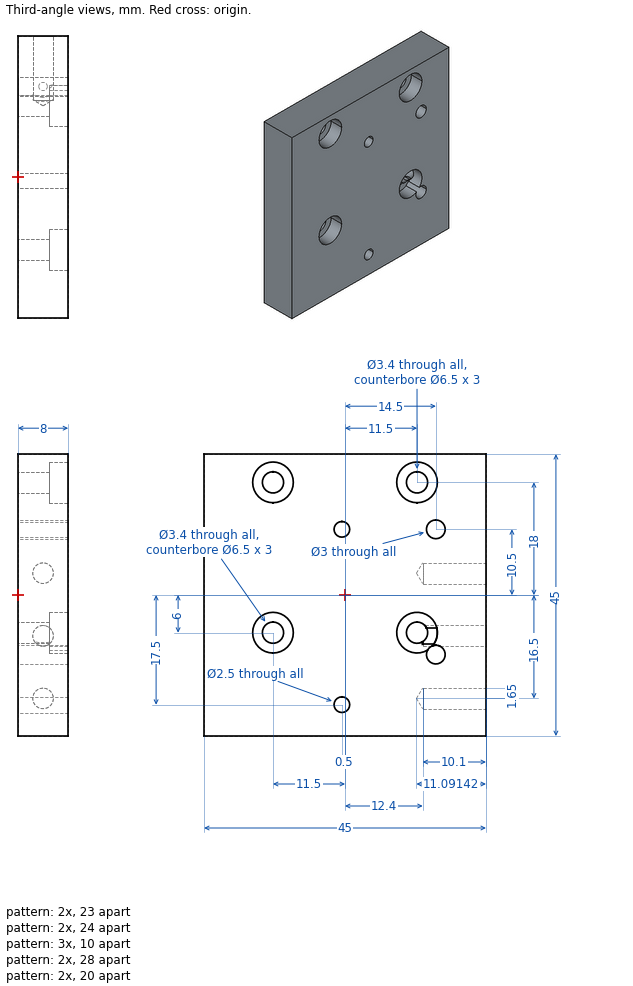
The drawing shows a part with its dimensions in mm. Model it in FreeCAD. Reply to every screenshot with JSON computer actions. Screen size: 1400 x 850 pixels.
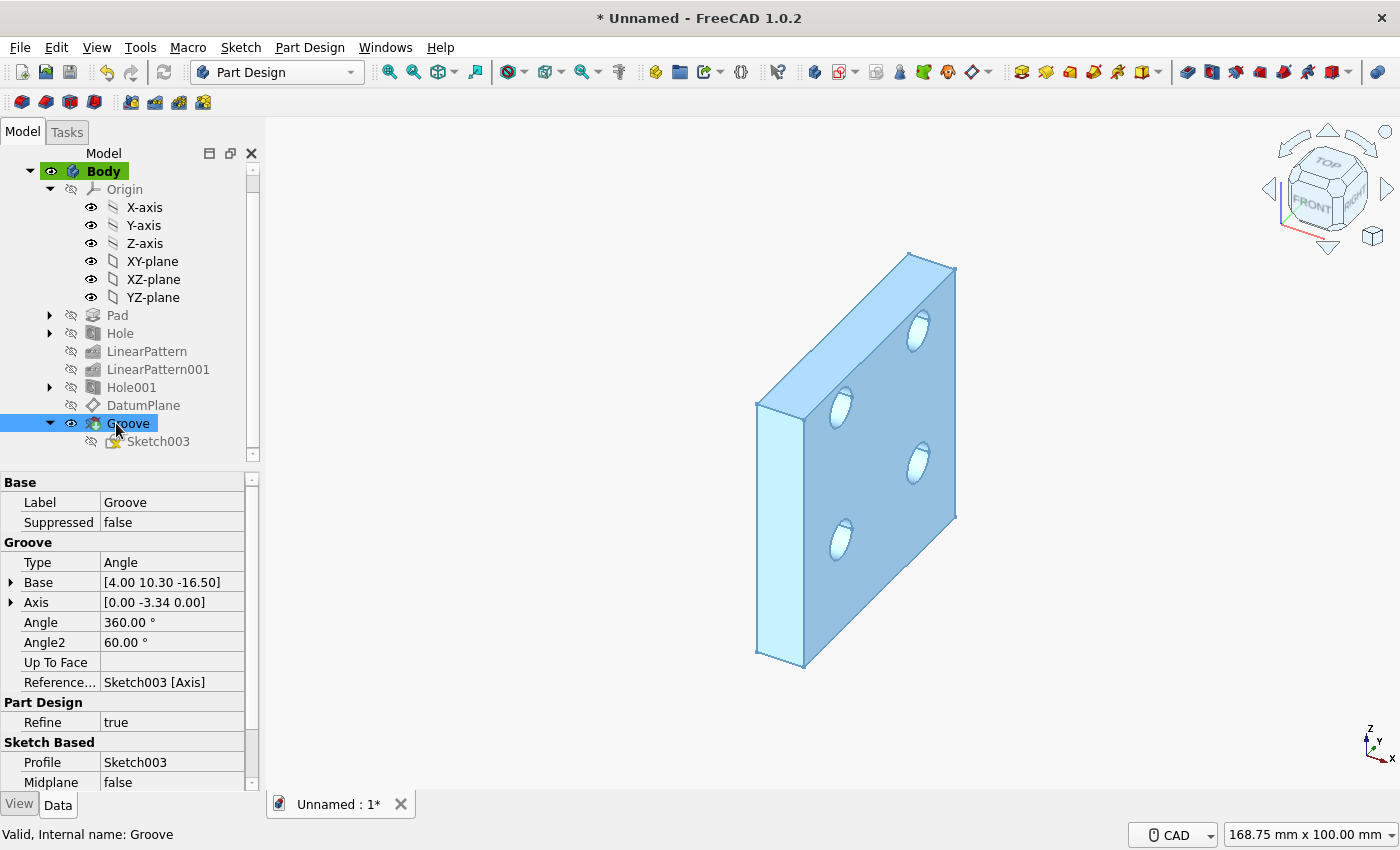
{"action": "left_click", "coordinate": [156, 102]}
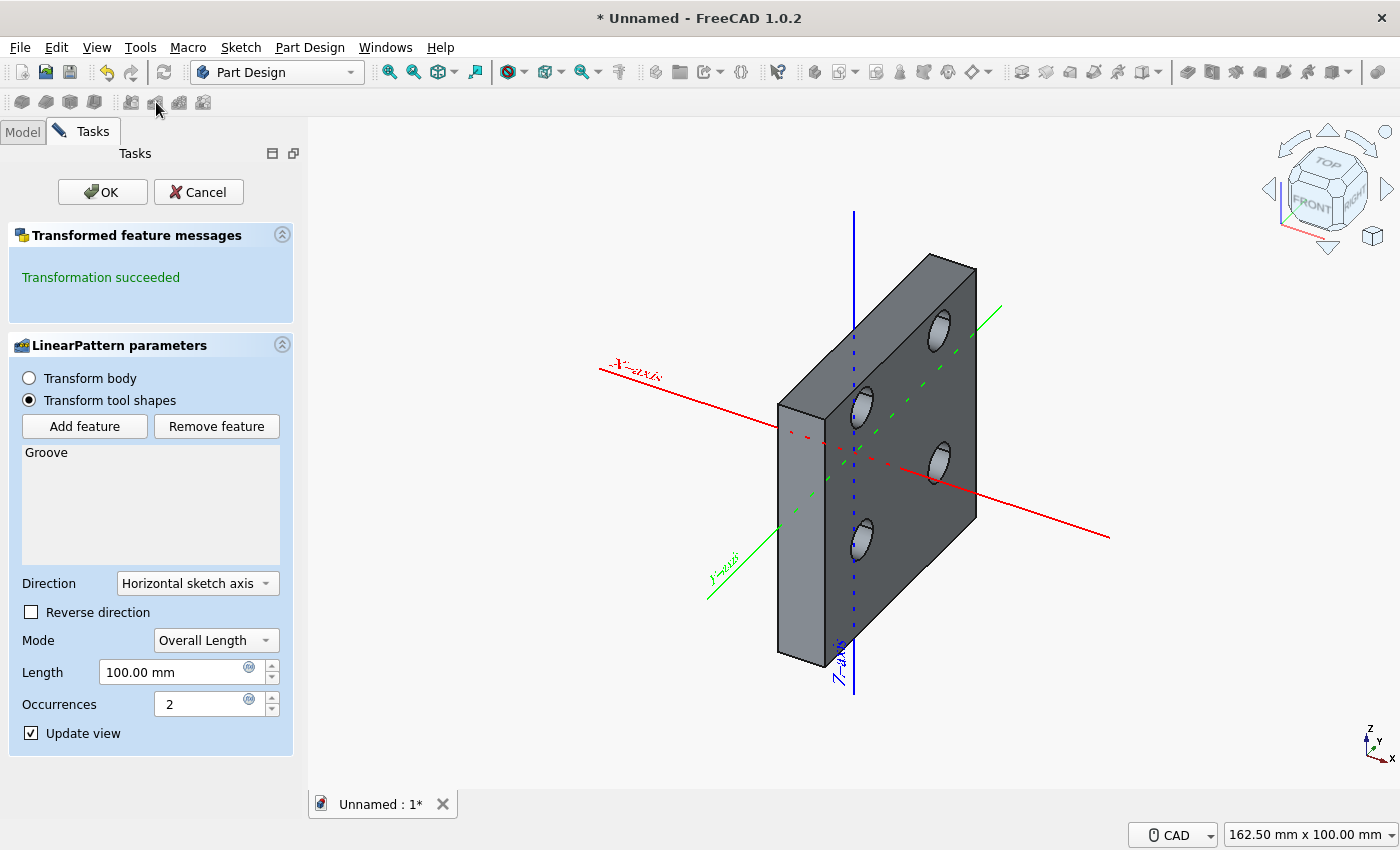
{"action": "left_click", "coordinate": [198, 584]}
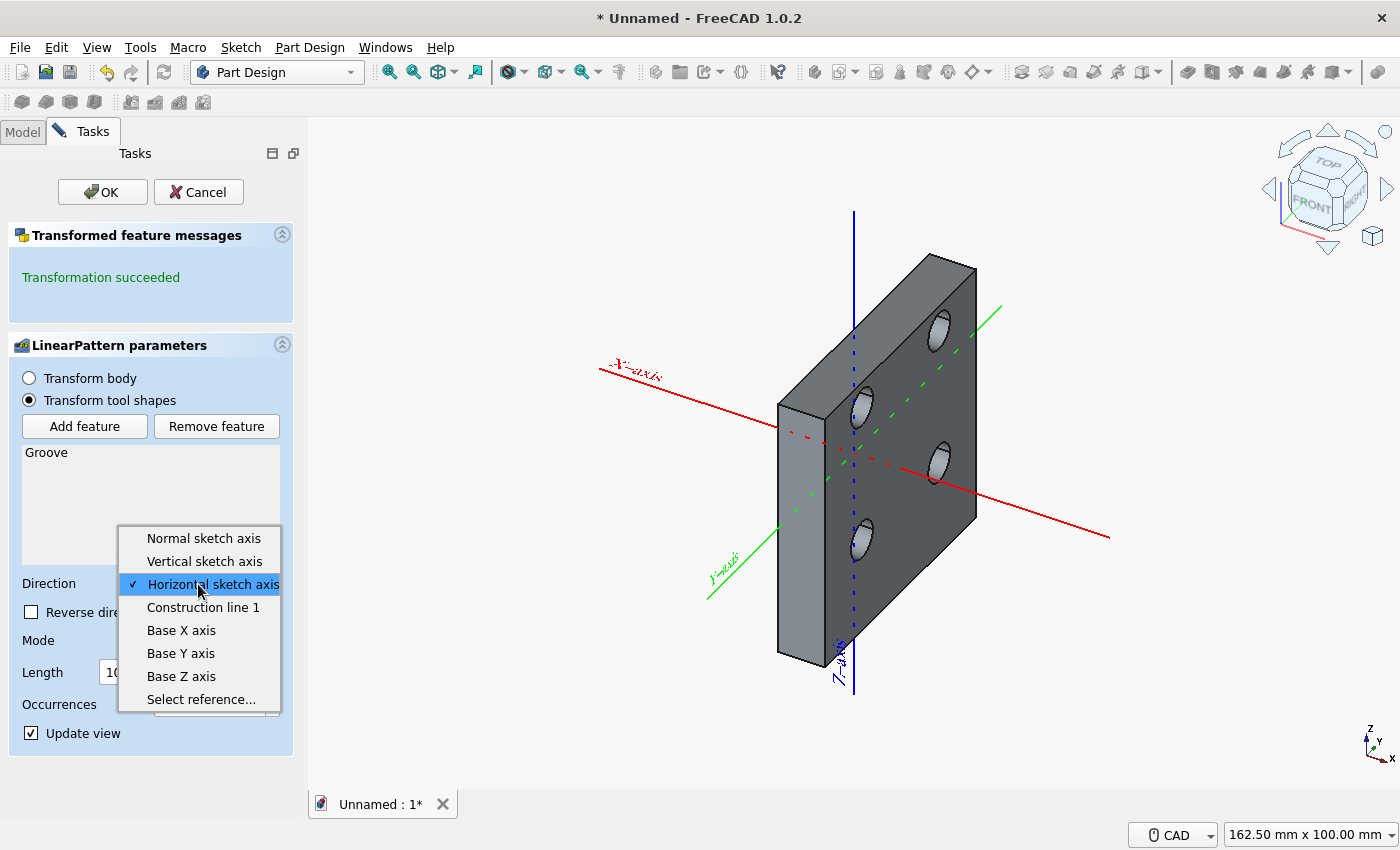
{"action": "left_click", "coordinate": [198, 676]}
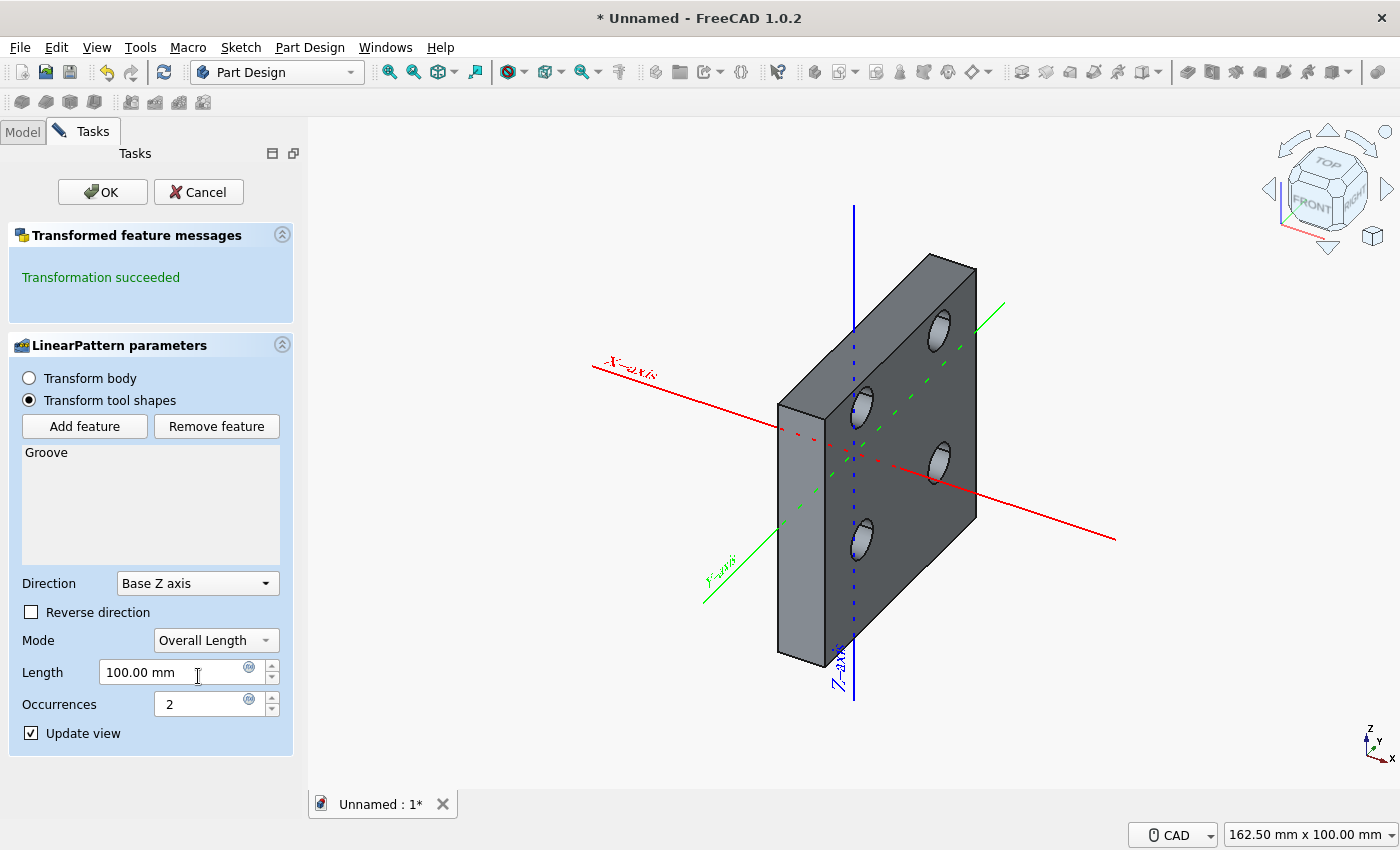
{"action": "left_click", "coordinate": [217, 640]}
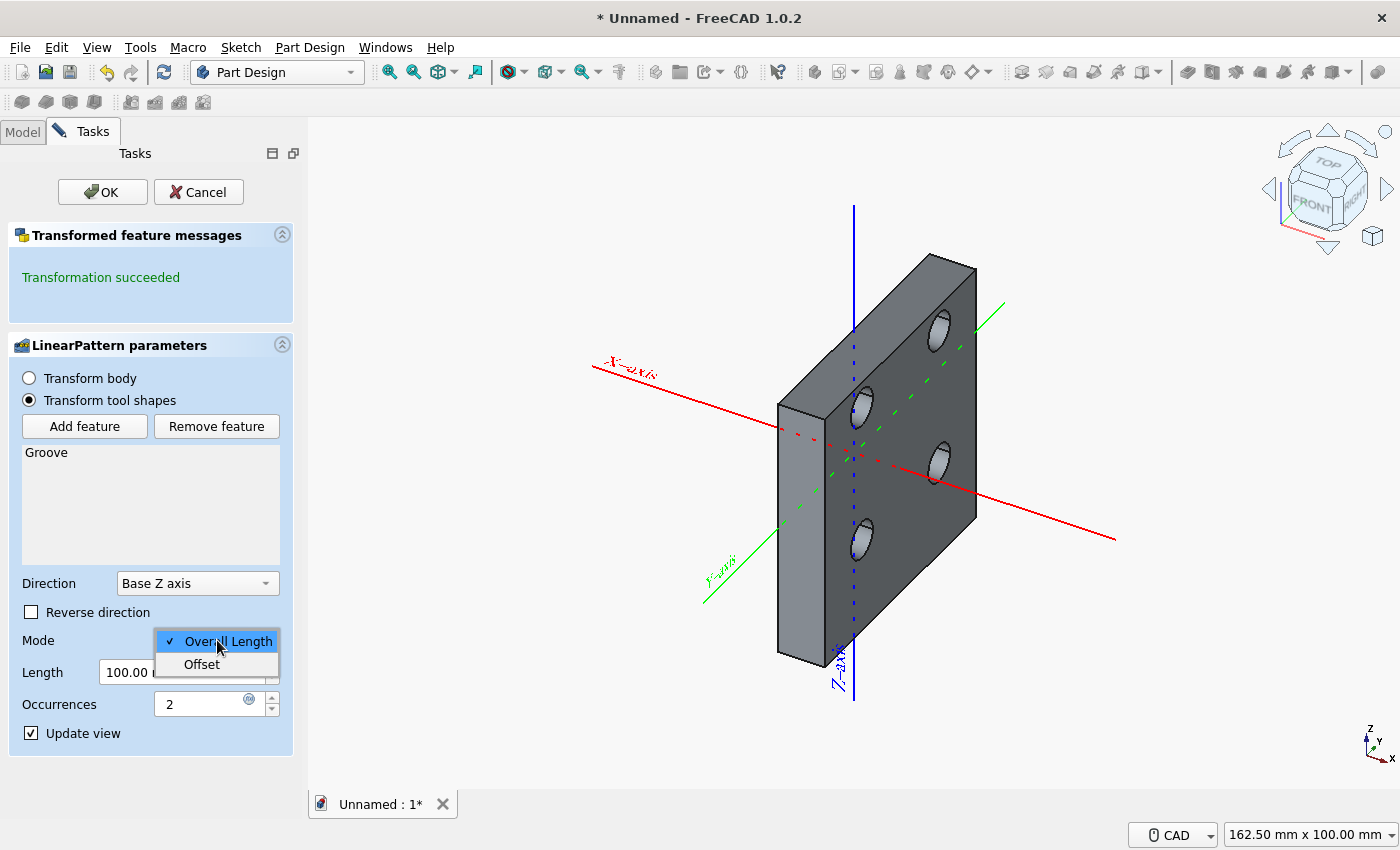
{"action": "left_click", "coordinate": [216, 664]}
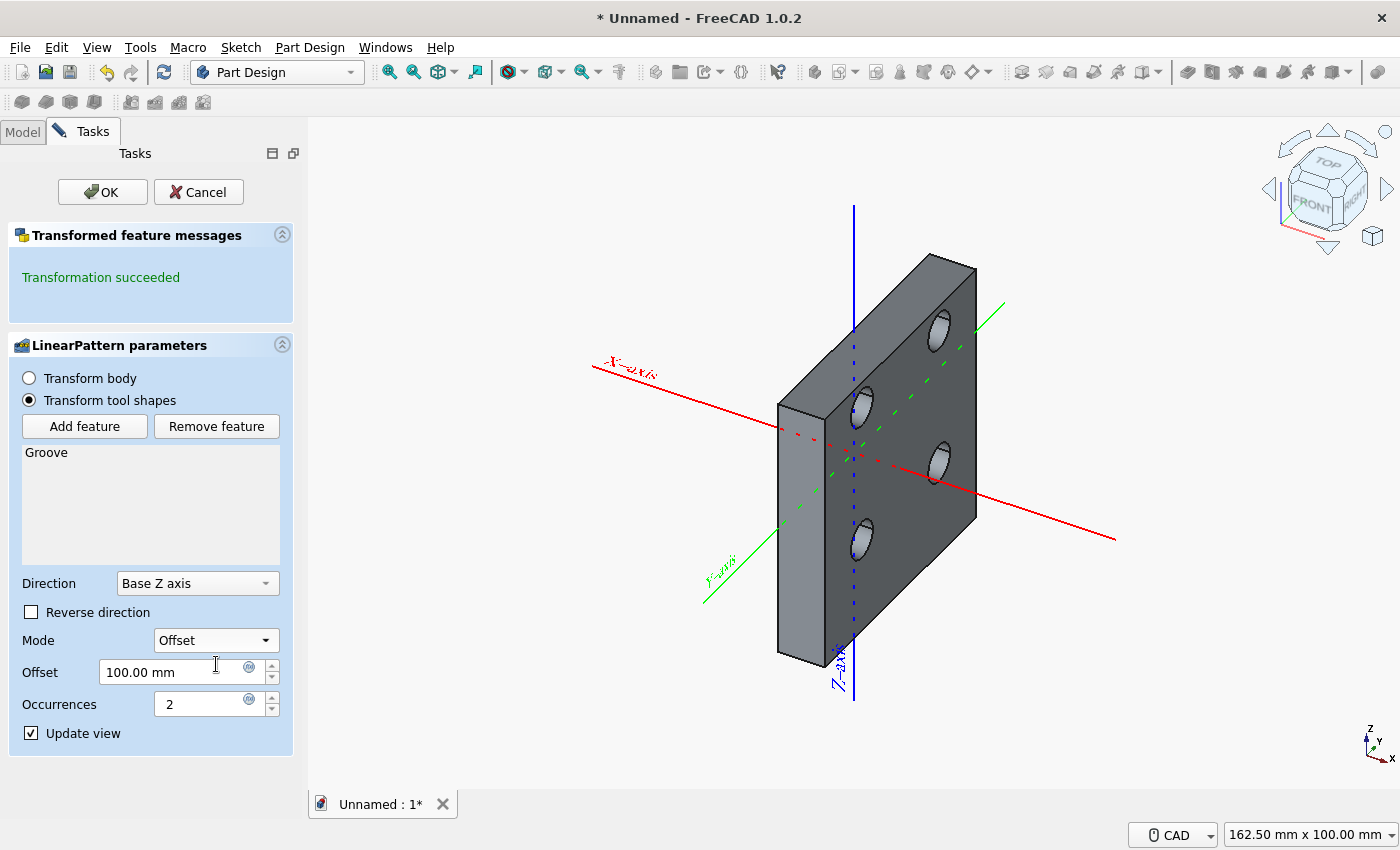
{"action": "triple_click", "coordinate": [182, 672]}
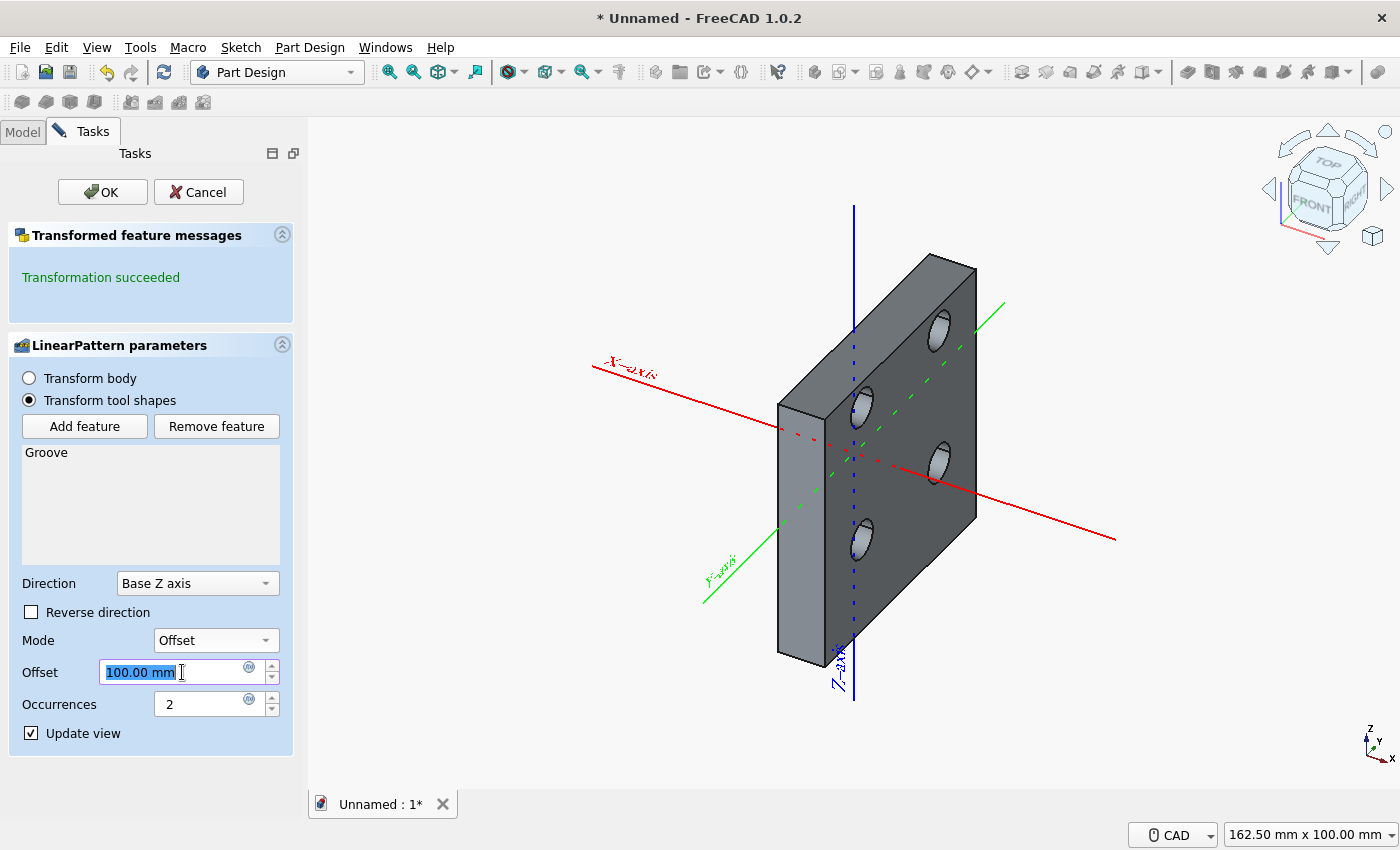
{"action": "type", "text": "10"}
{"action": "key", "text": "Tab"}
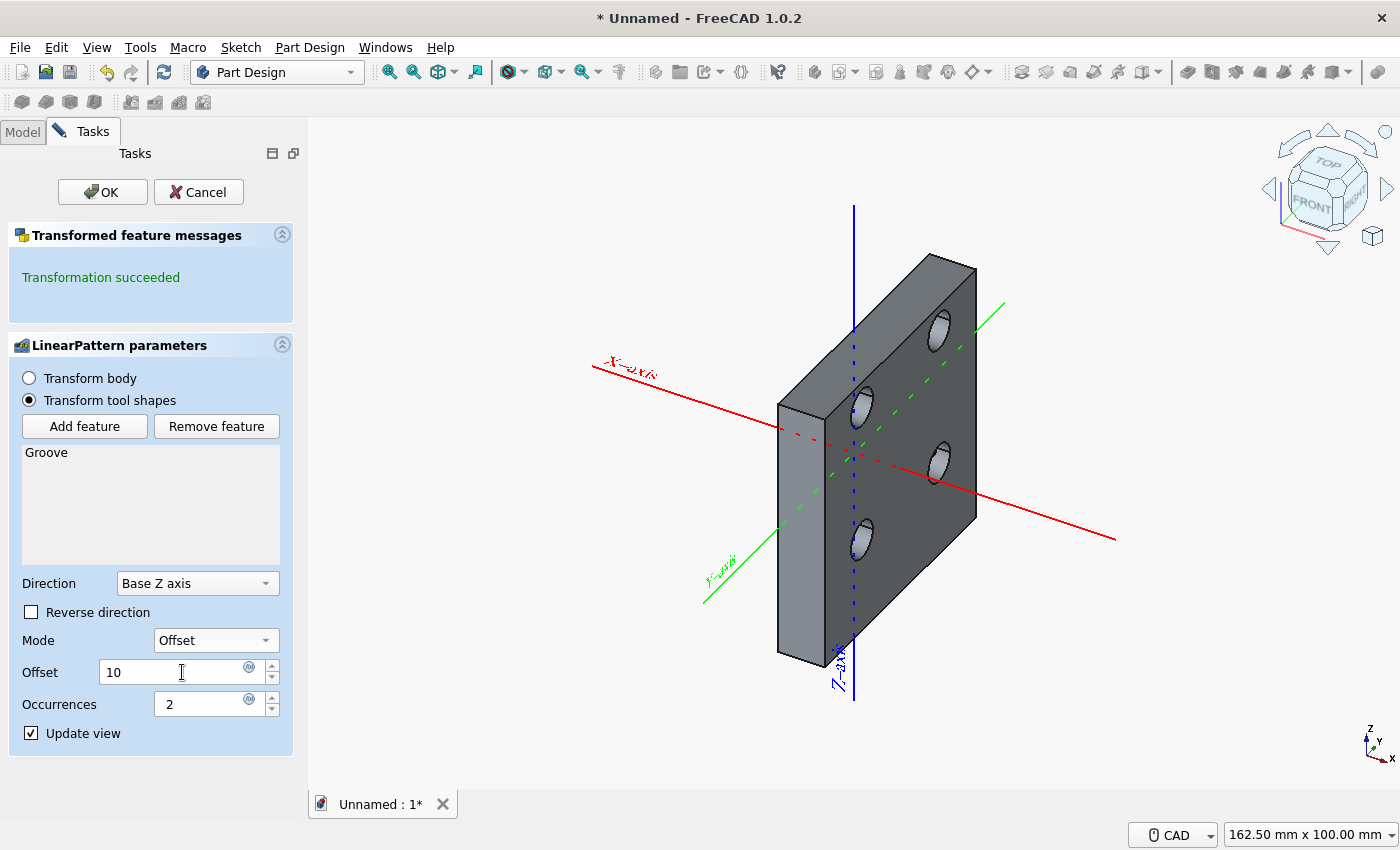
{"action": "triple_click", "coordinate": [209, 704]}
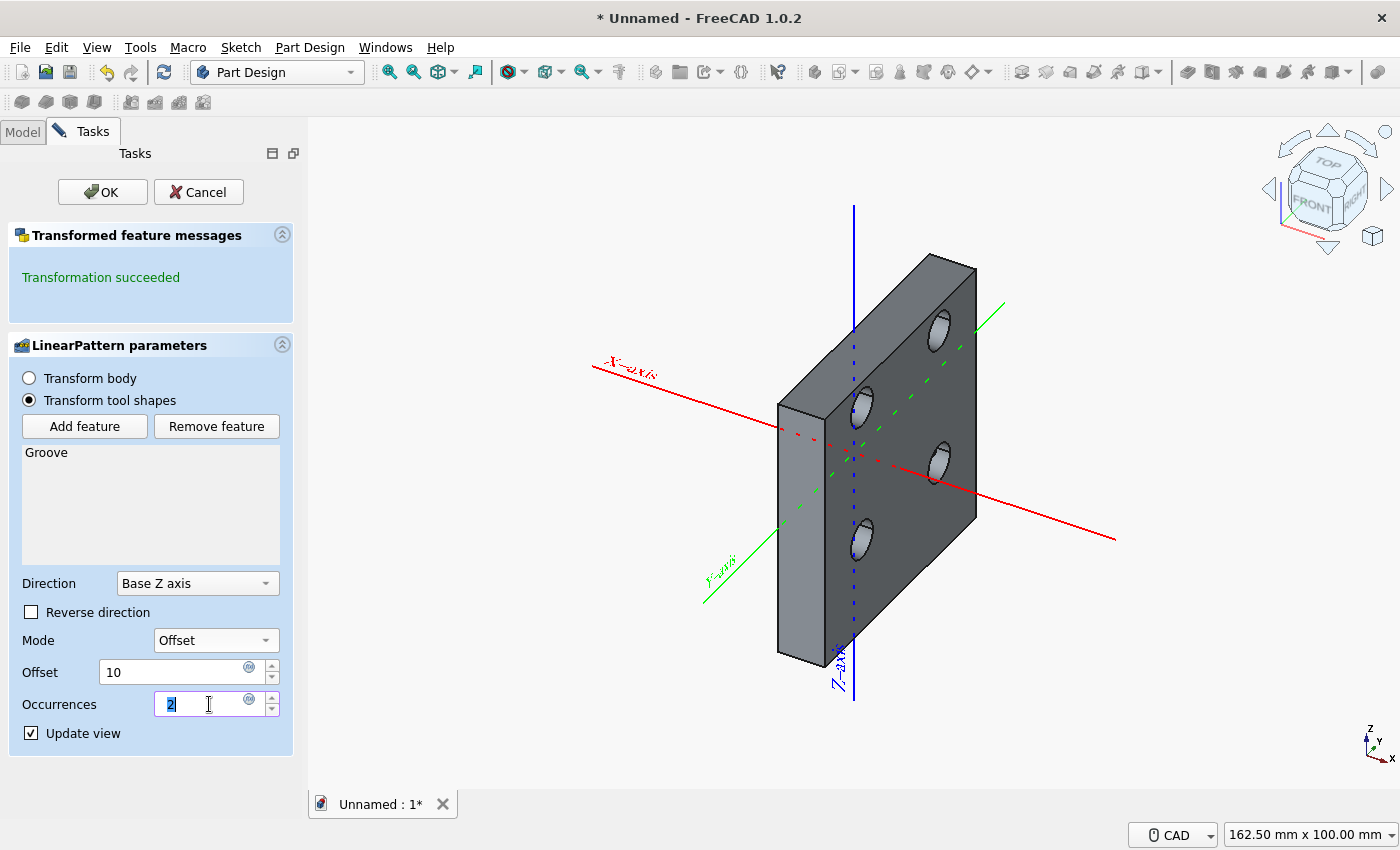
{"action": "type", "text": "3"}
{"action": "key", "text": "Tab"}